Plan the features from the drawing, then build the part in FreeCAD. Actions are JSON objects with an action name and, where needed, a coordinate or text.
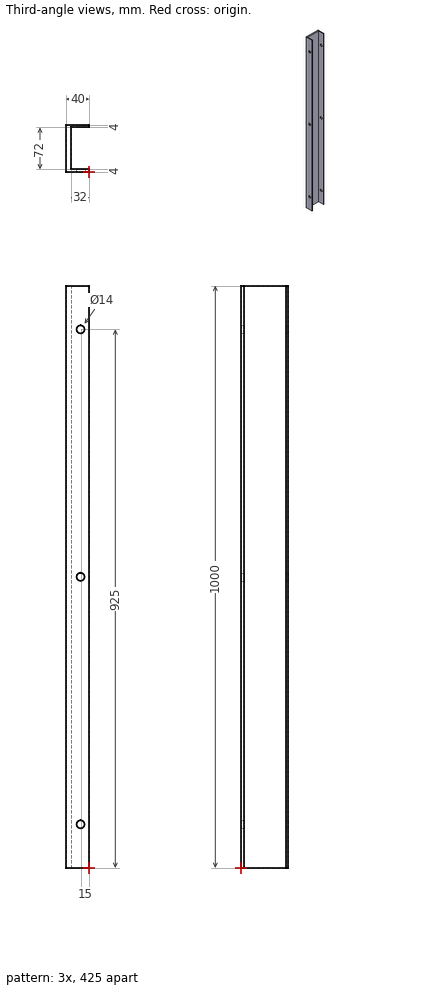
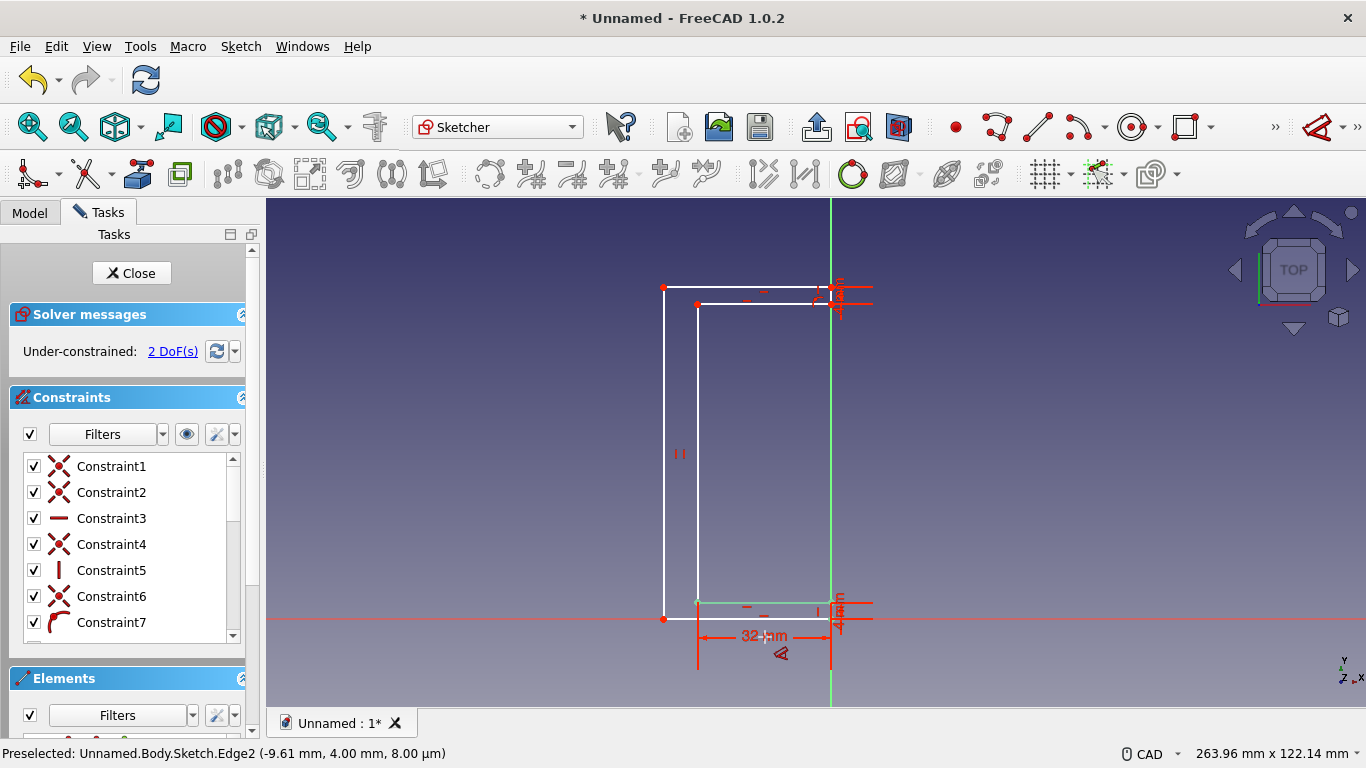
{"action": "left_click", "coordinate": [698, 513]}
{"action": "left_click", "coordinate": [732, 453]}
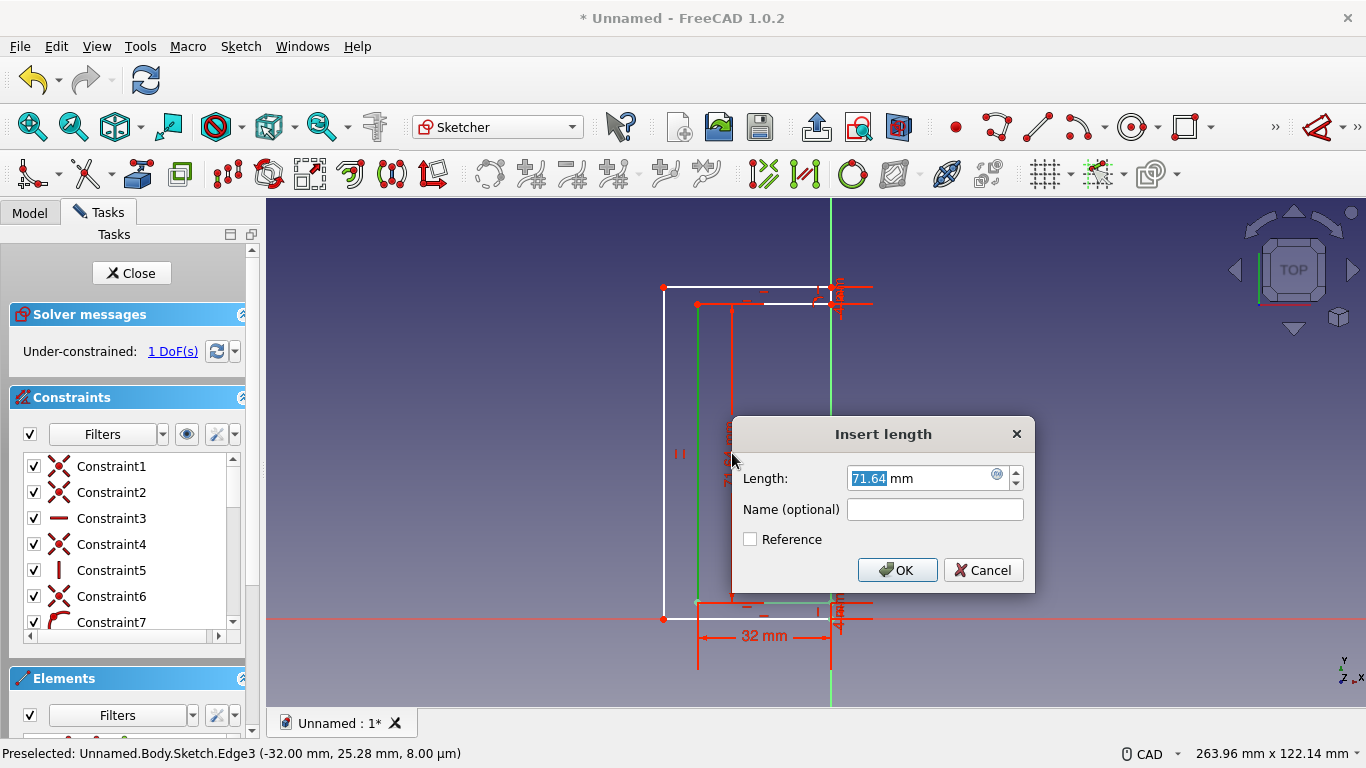
{"action": "type", "text": "72"}
{"action": "key", "text": "Return"}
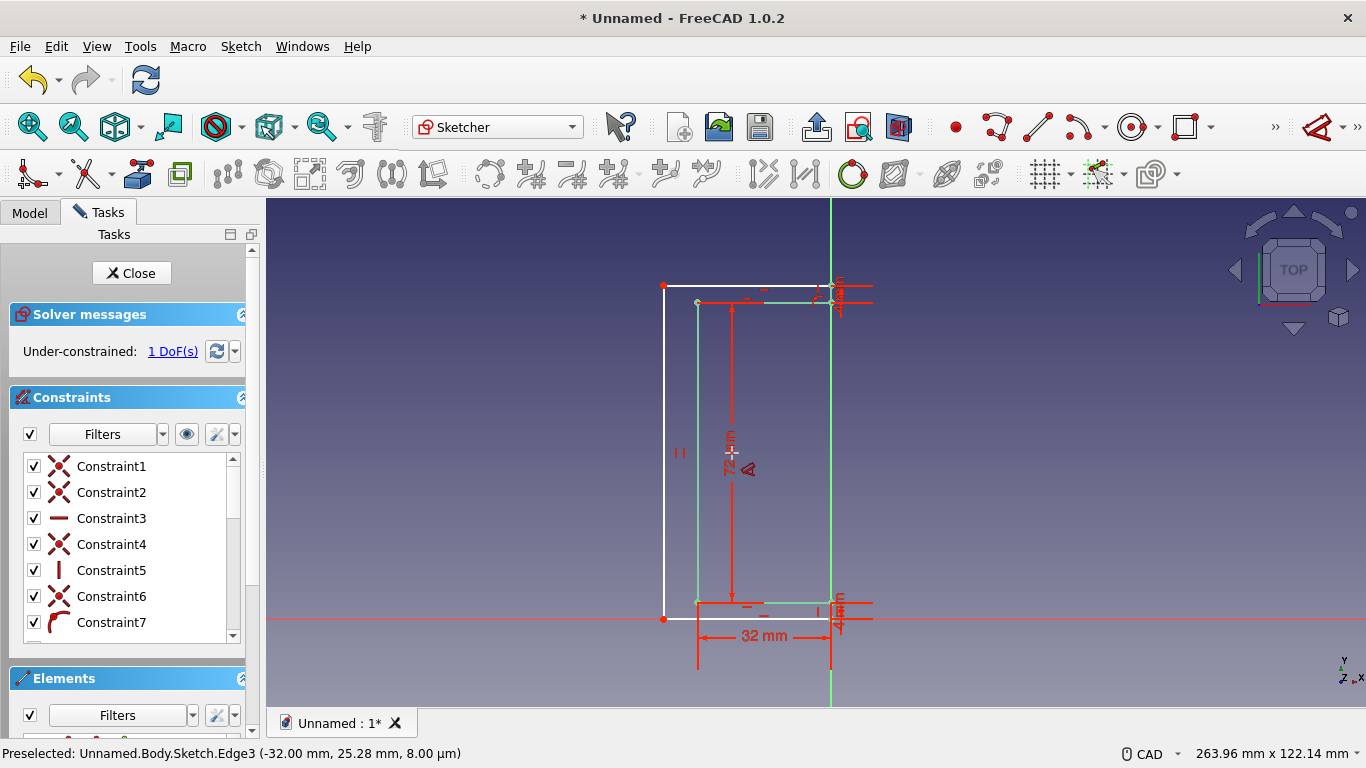
{"action": "left_click", "coordinate": [781, 286]}
{"action": "left_click", "coordinate": [747, 252]}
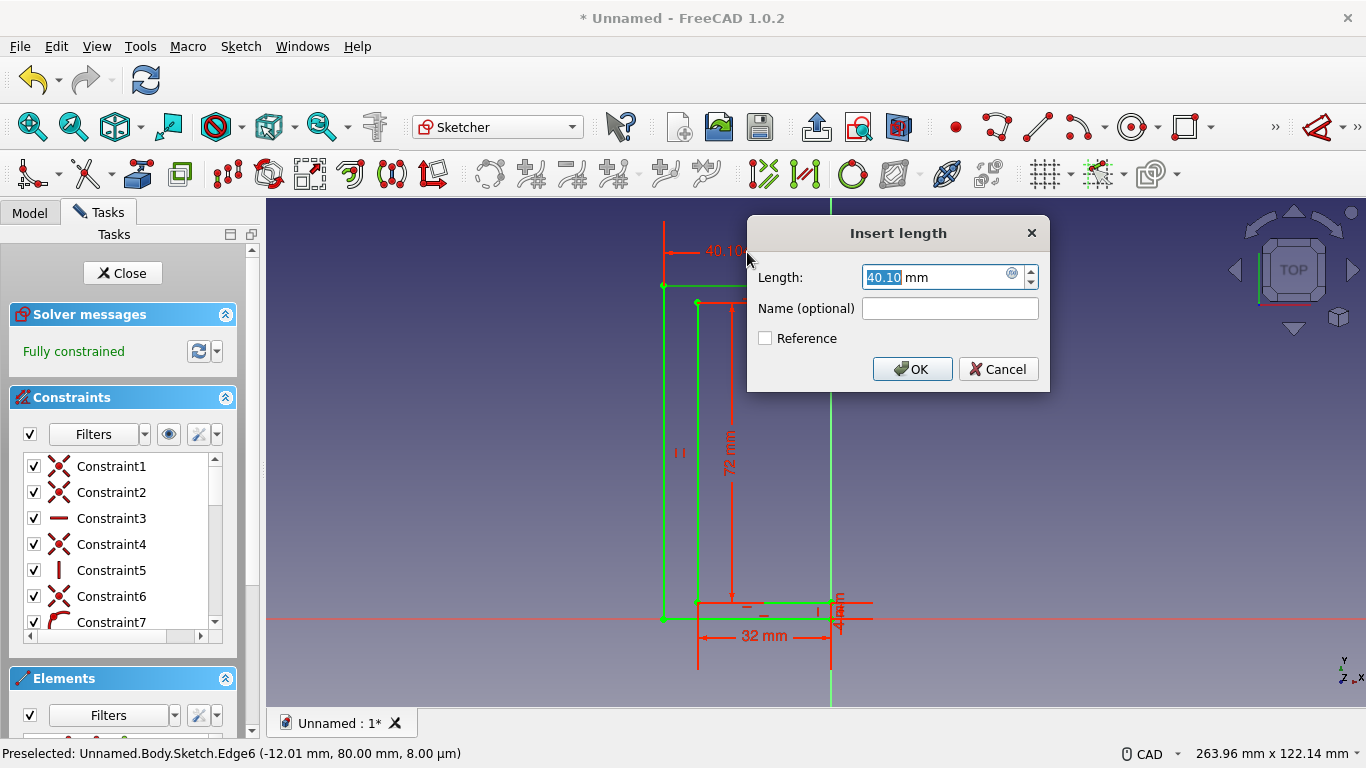
{"action": "type", "text": "40"}
{"action": "key", "text": "Return"}
{"action": "key", "text": "Escape"}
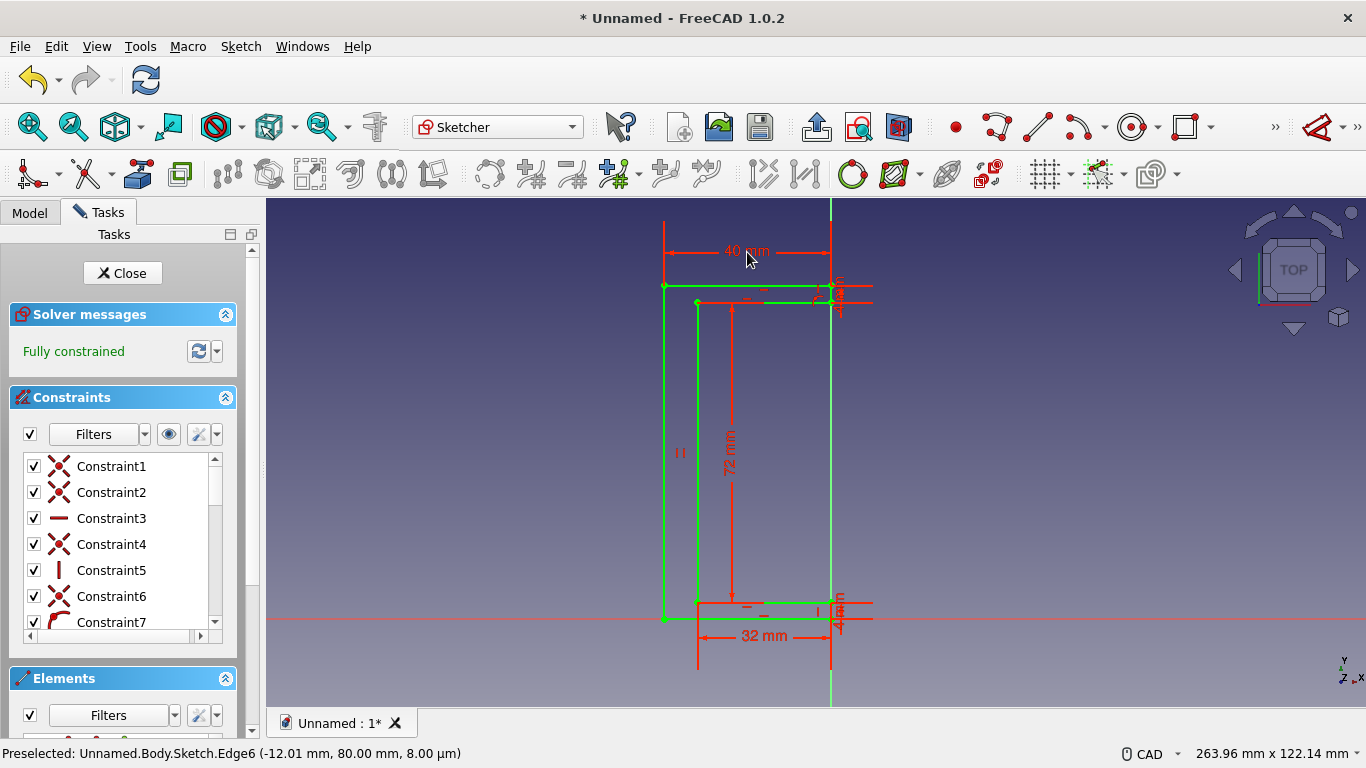
{"action": "left_click", "coordinate": [123, 273]}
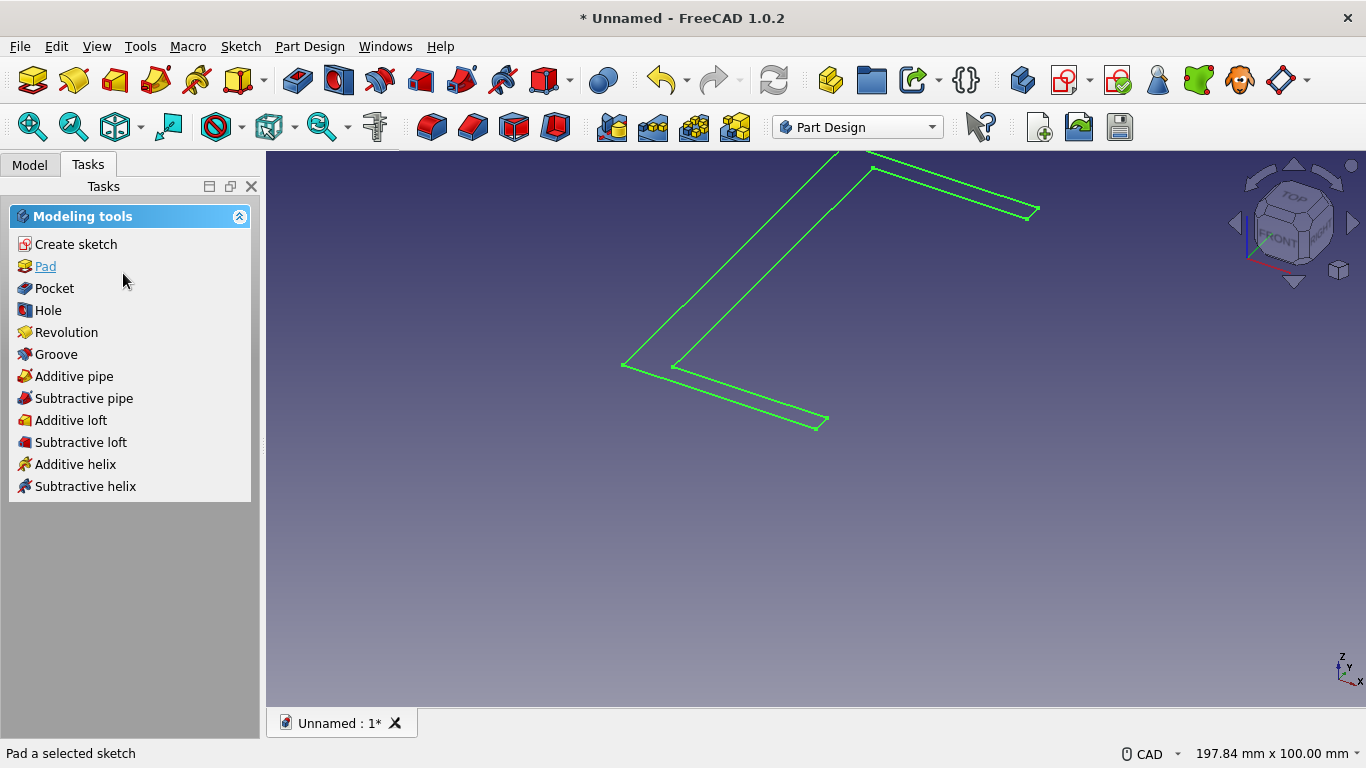
{"action": "left_click", "coordinate": [33, 80]}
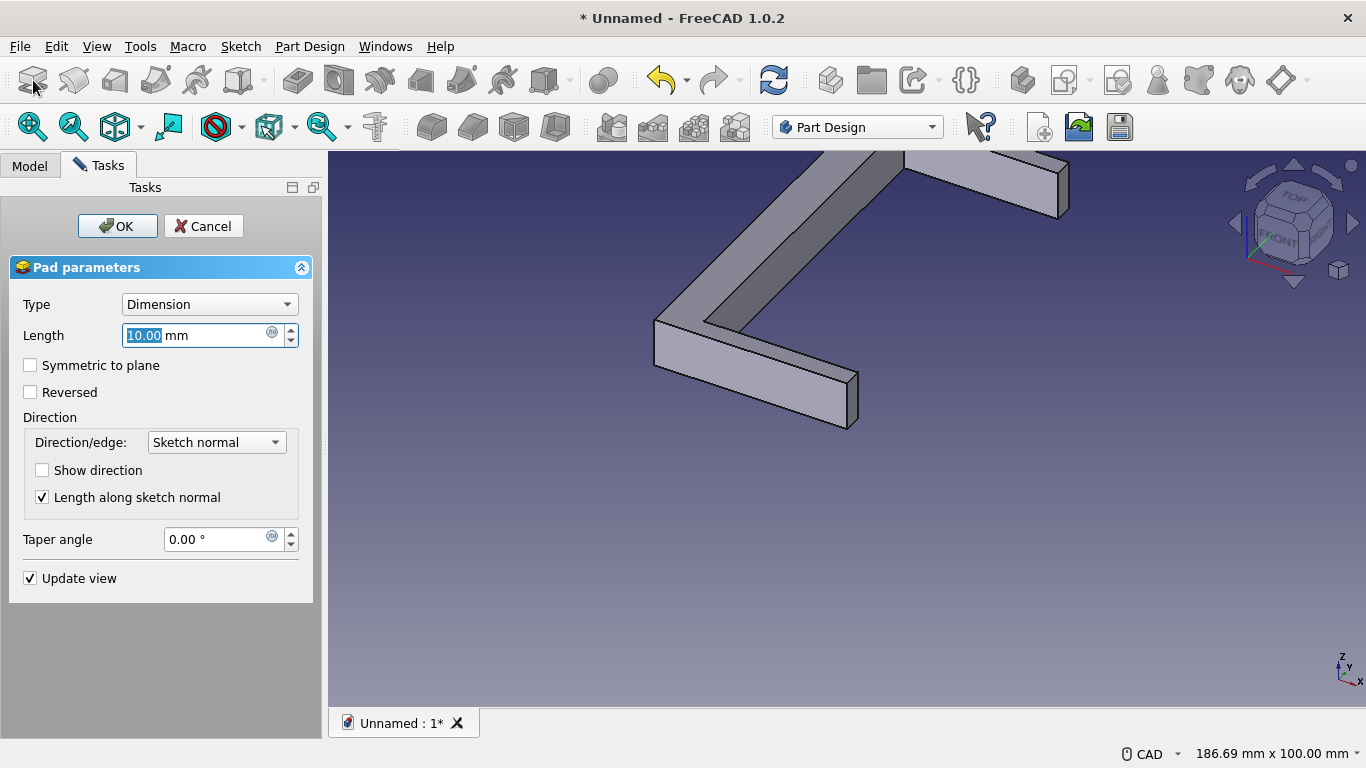
{"action": "type", "text": "1000"}
{"action": "key", "text": "Tab"}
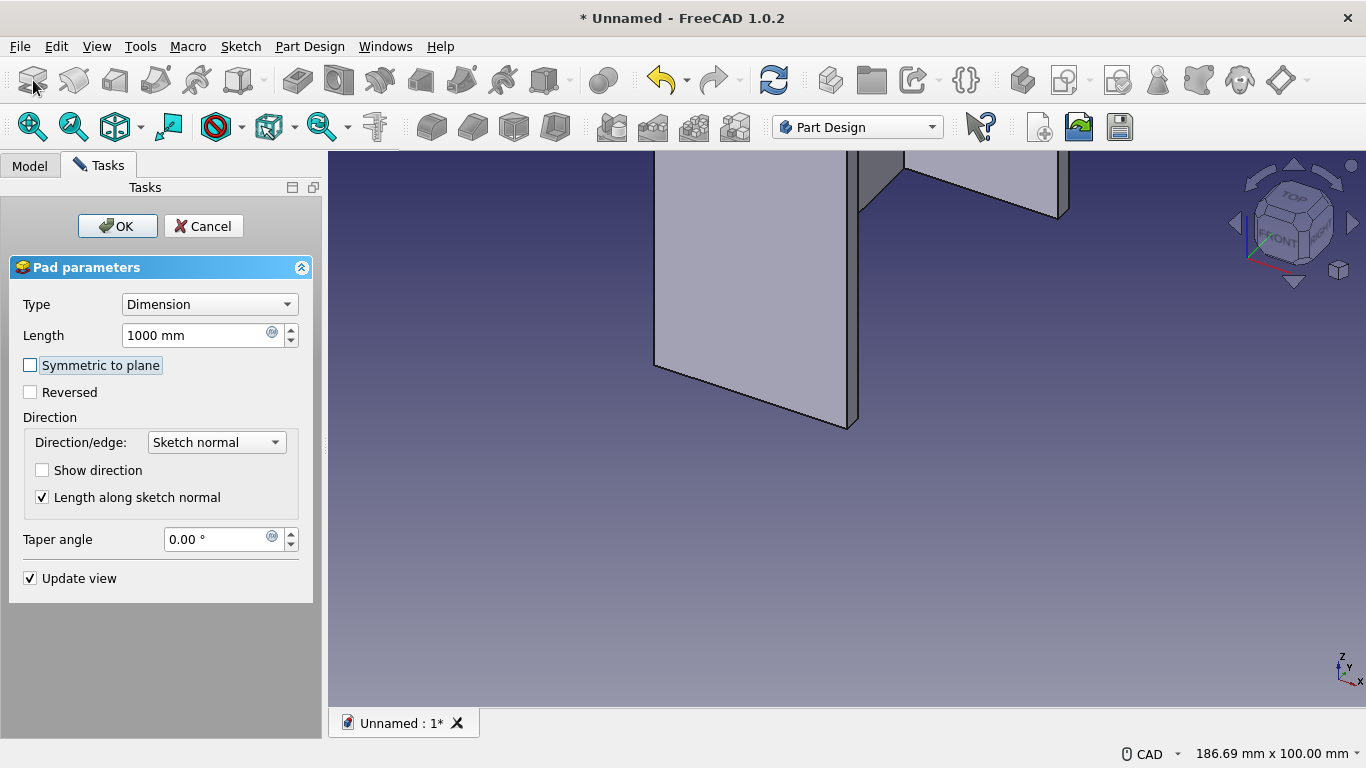
{"action": "left_click", "coordinate": [118, 226]}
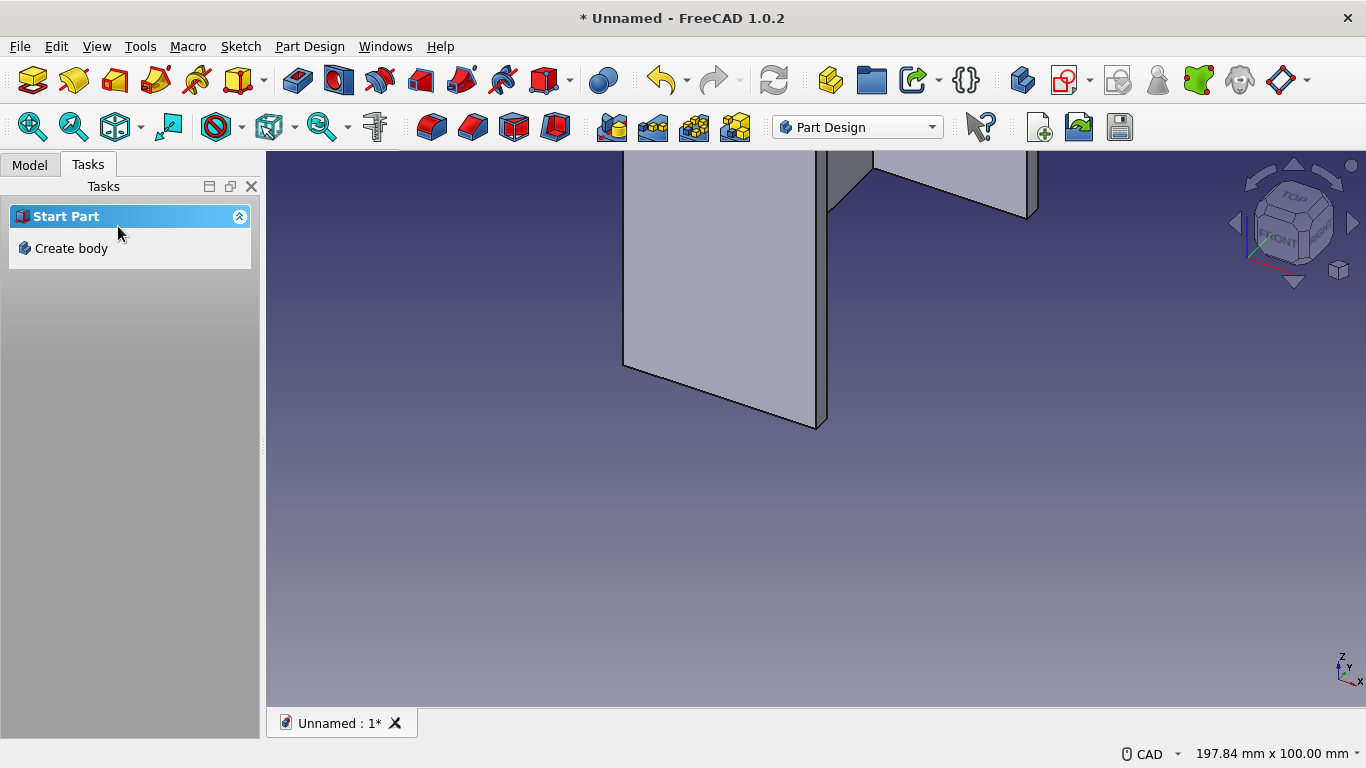
{"action": "left_click", "coordinate": [33, 128]}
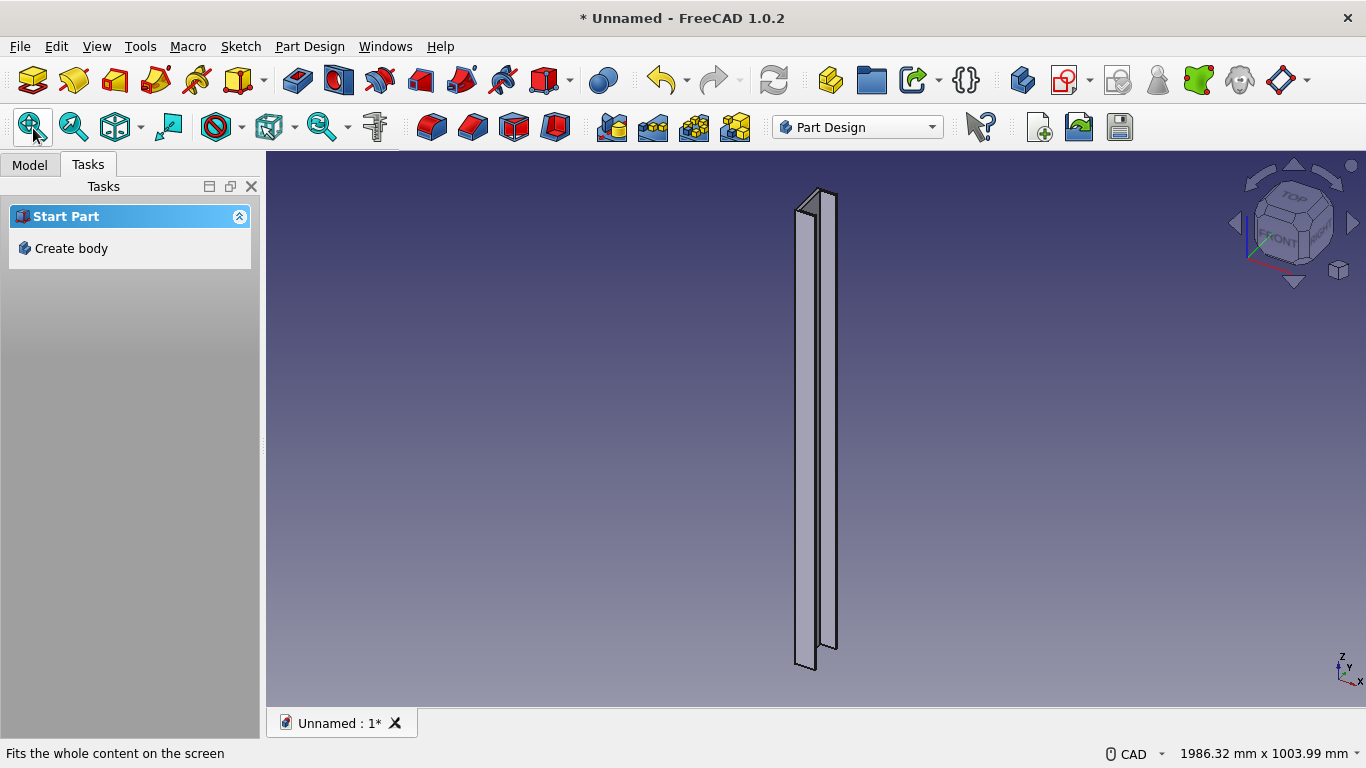
{"action": "key", "text": "4"}